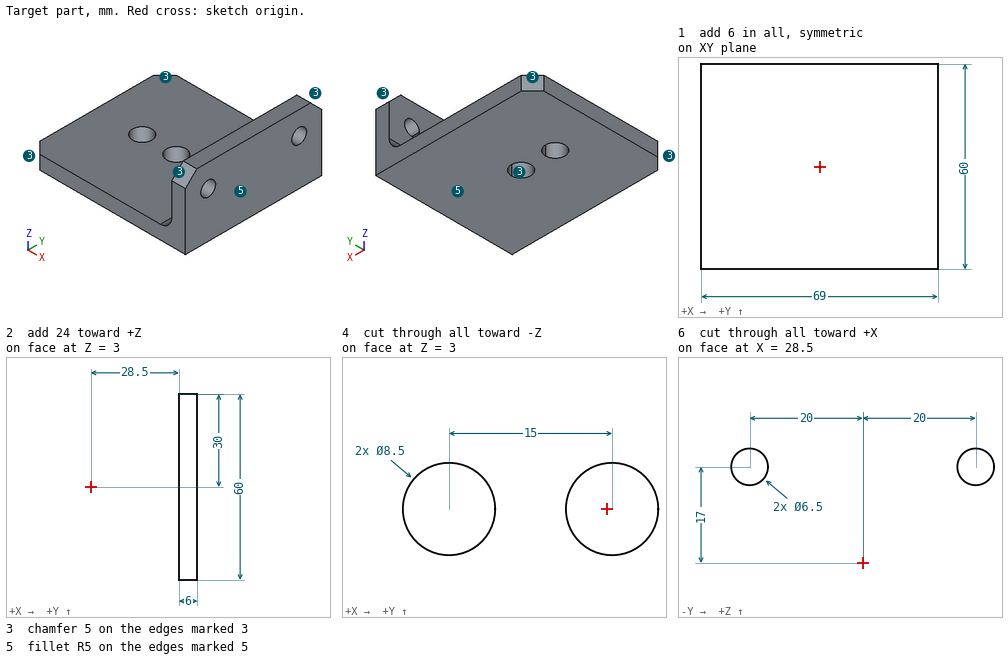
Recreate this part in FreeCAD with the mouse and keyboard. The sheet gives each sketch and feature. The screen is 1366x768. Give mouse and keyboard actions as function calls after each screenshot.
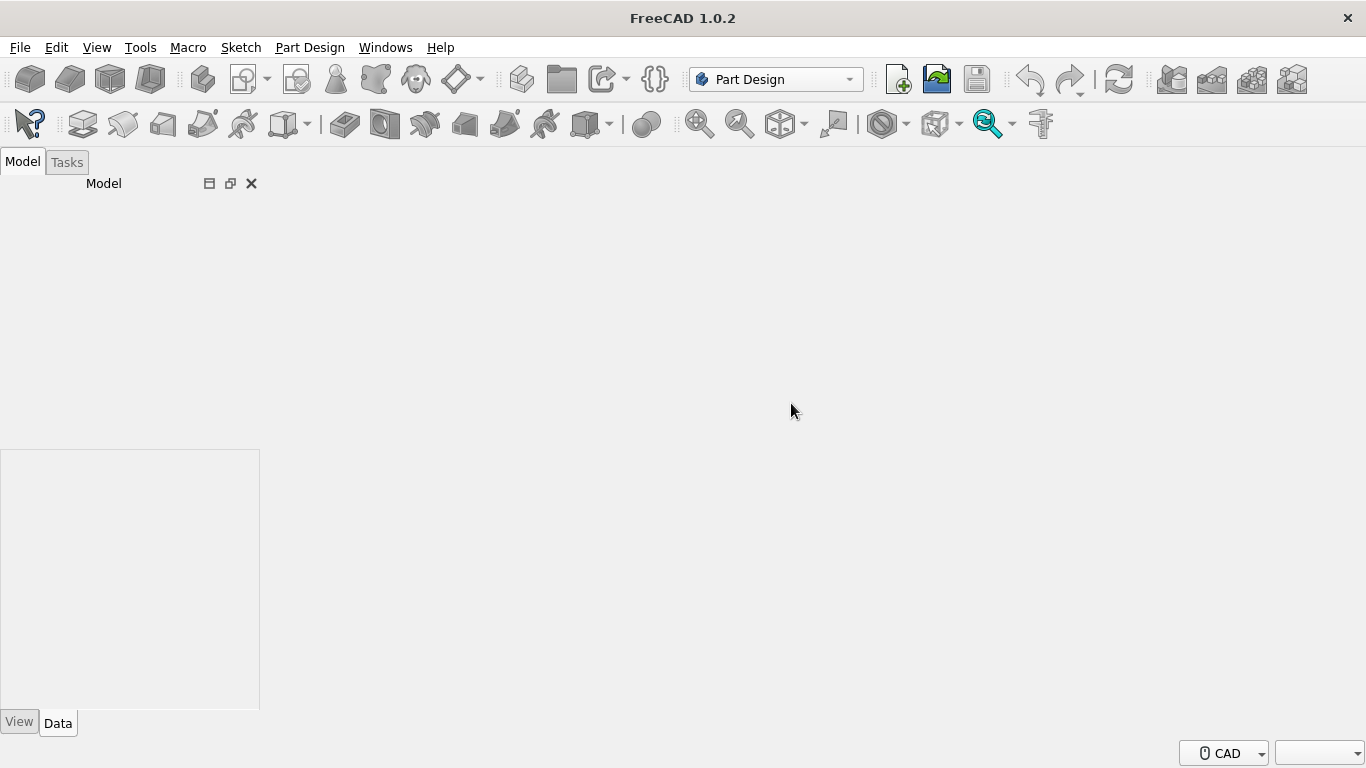
key(ctrl+n)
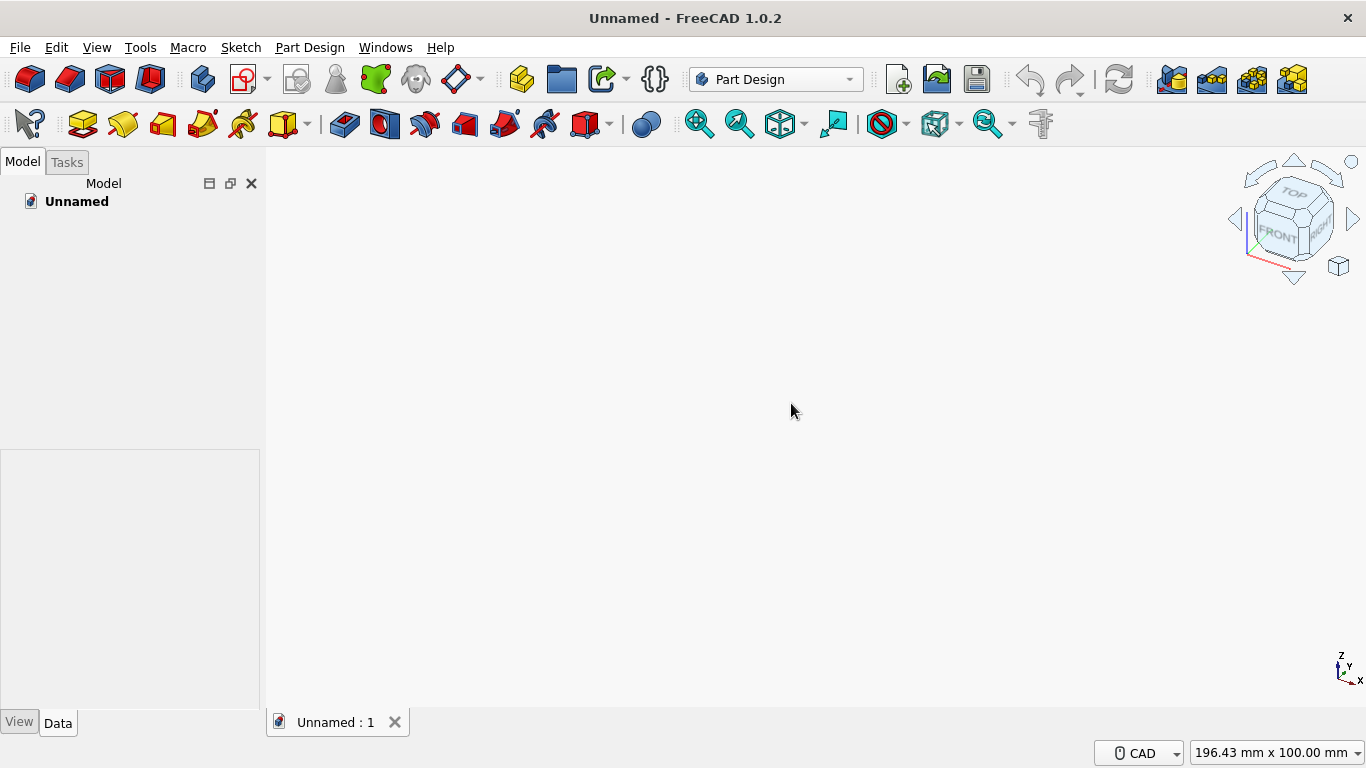
click(244, 80)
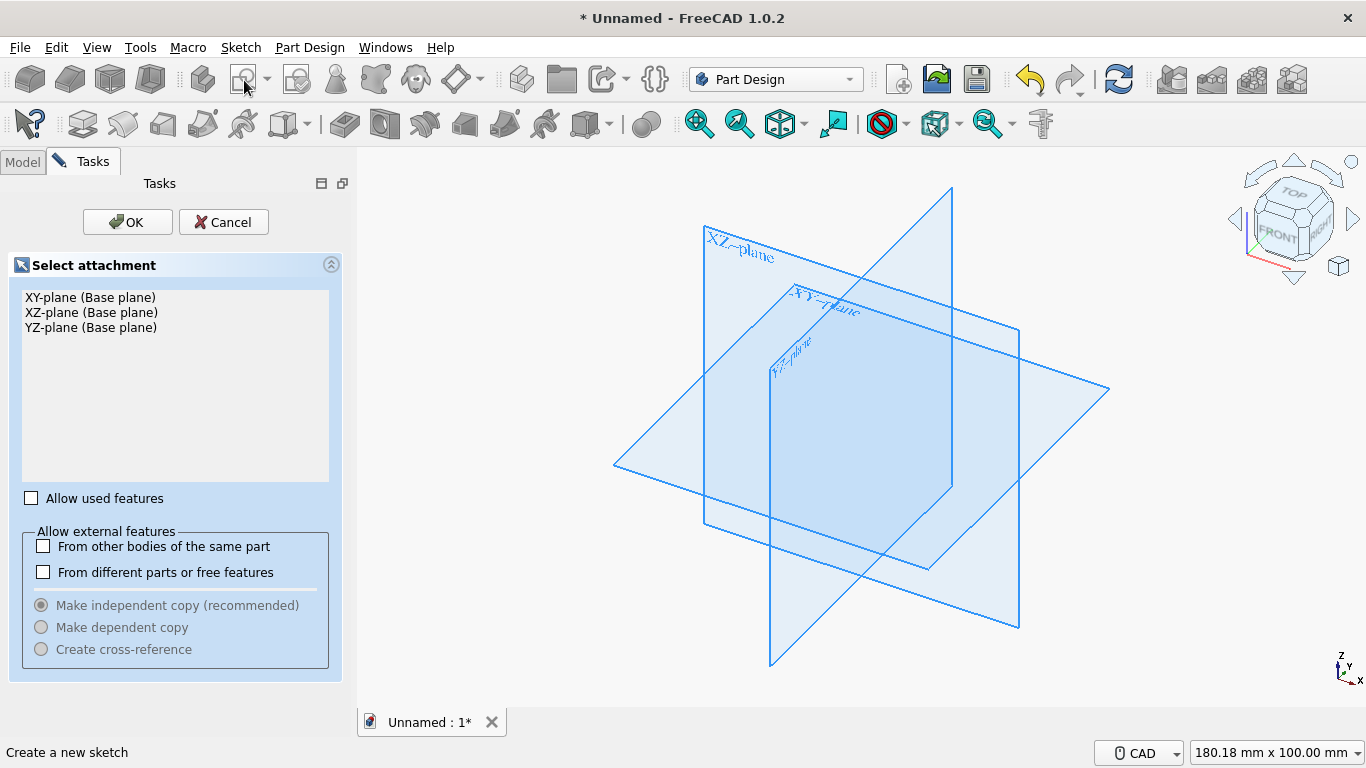
click(82, 298)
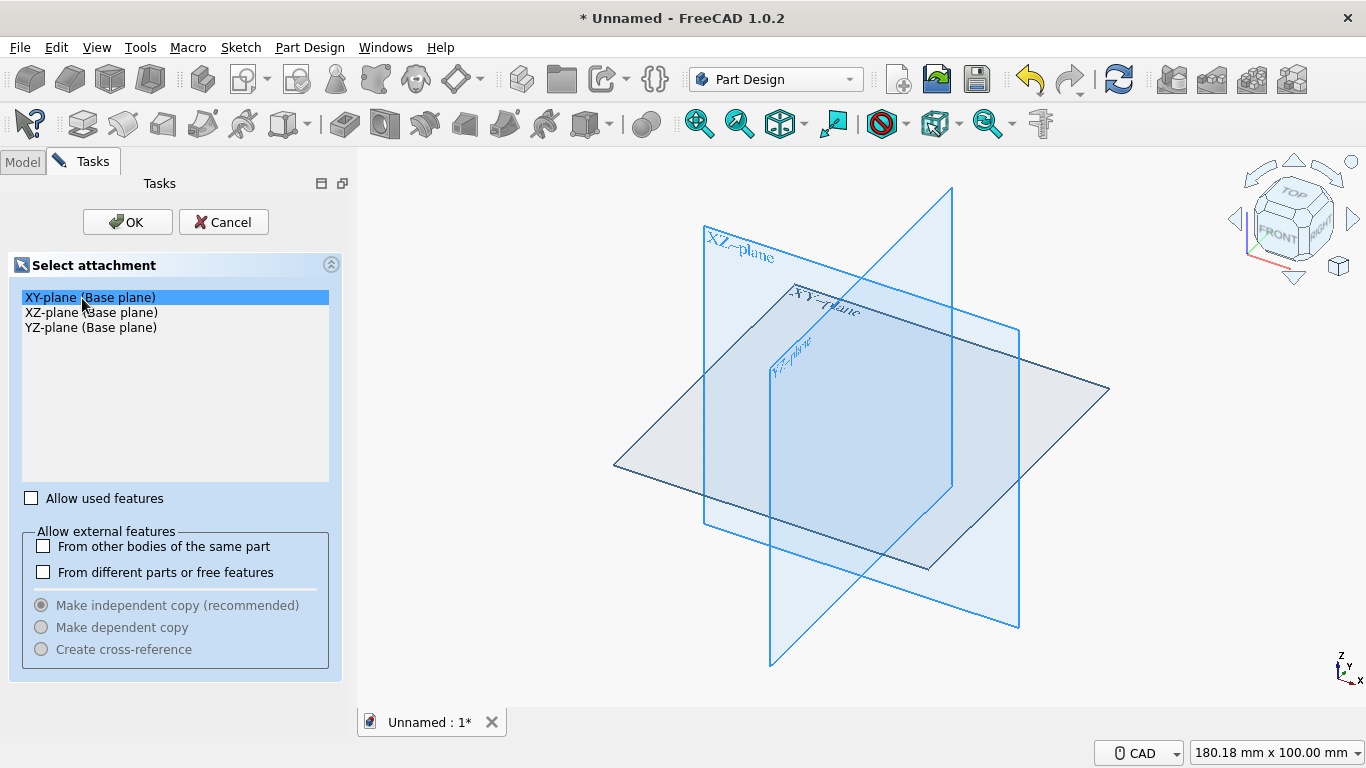
click(128, 222)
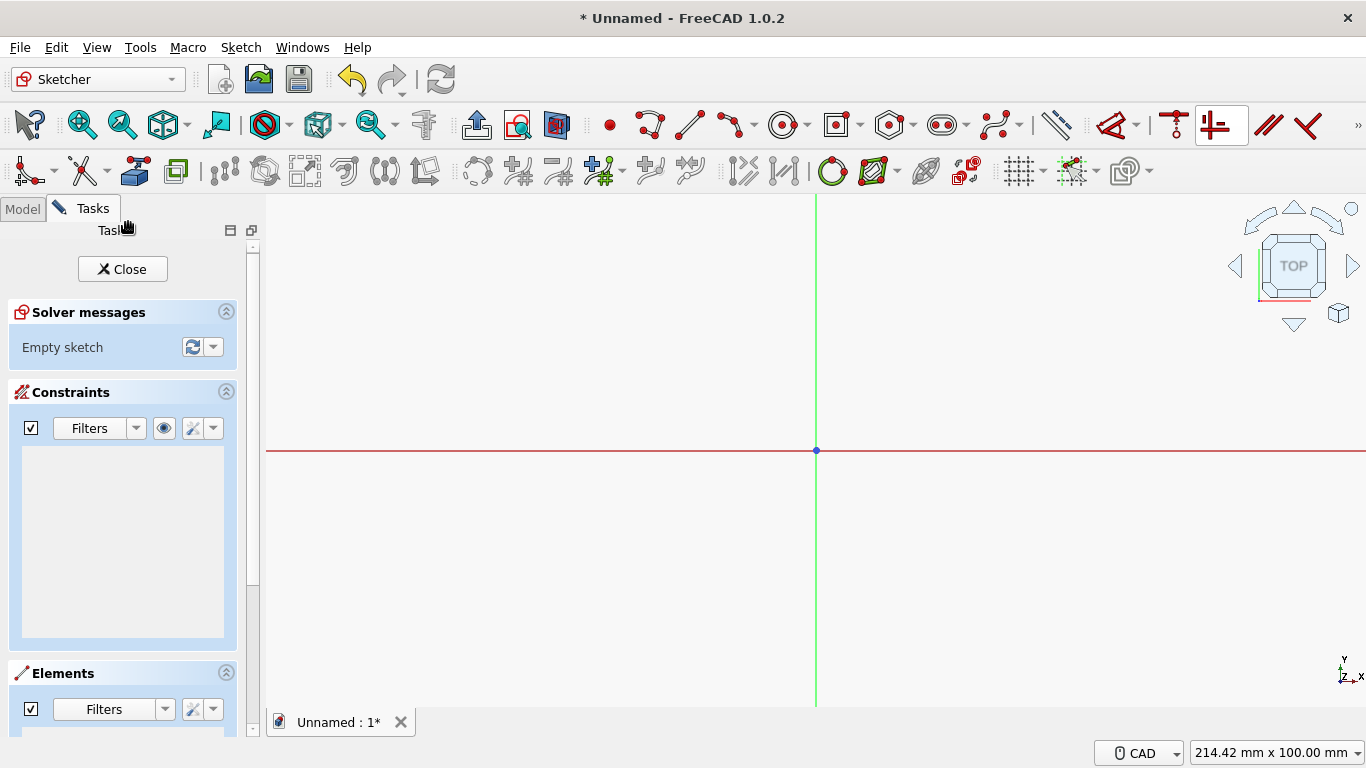
click(836, 126)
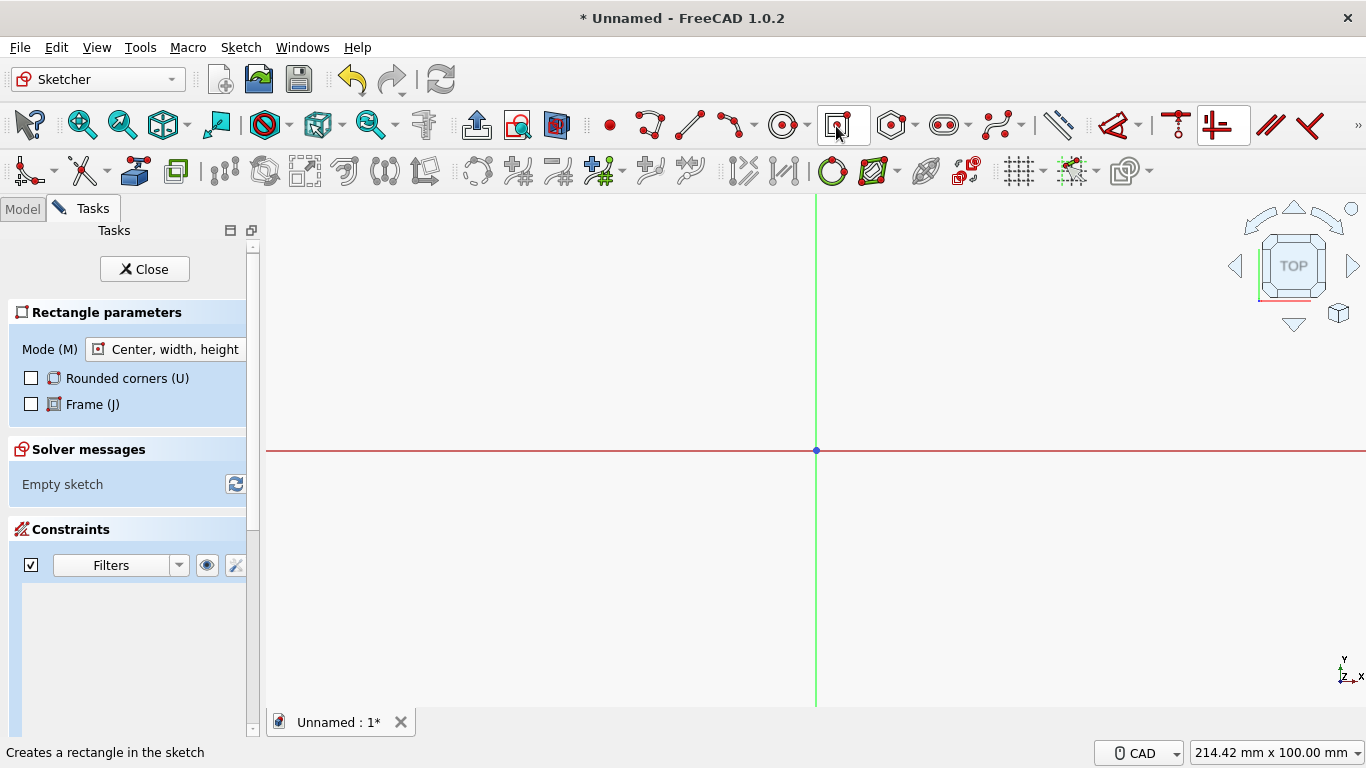
click(816, 450)
move(993, 297)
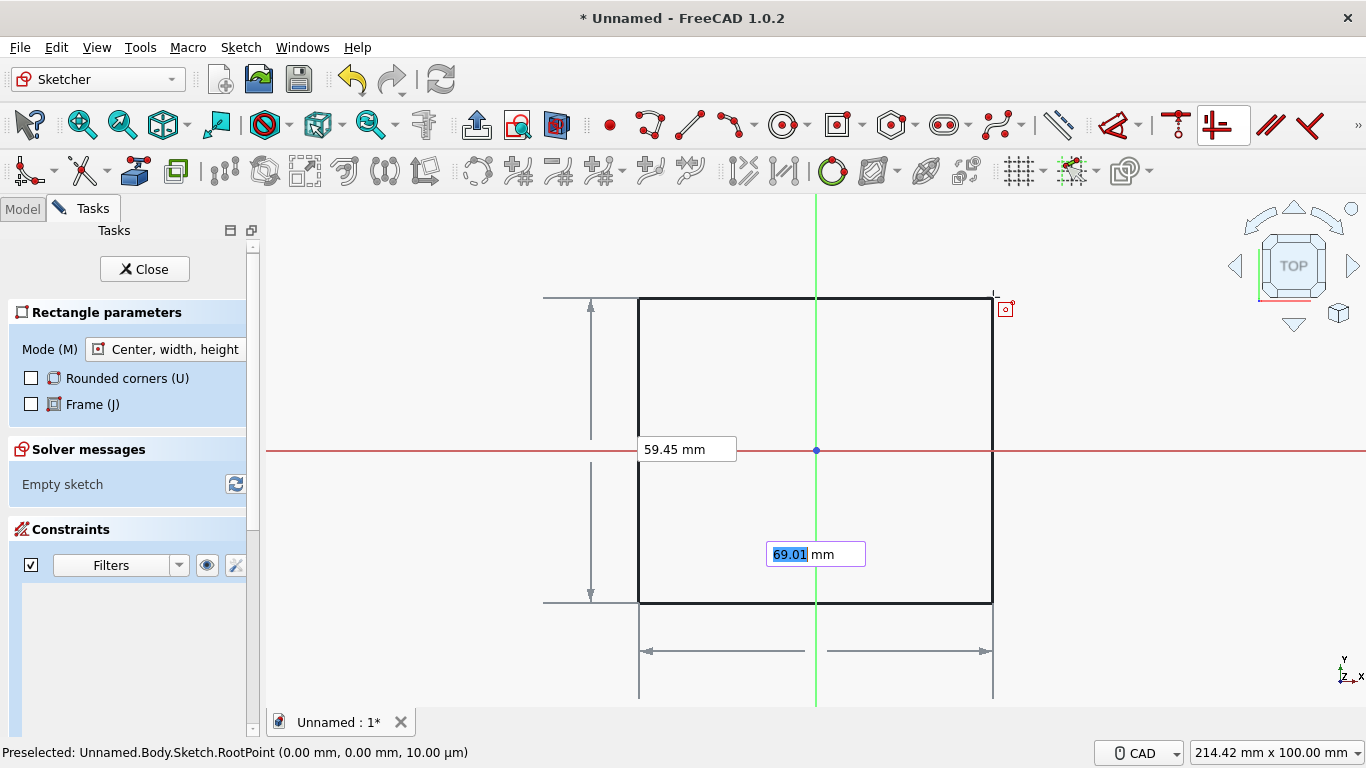
text(69)
key(Tab)
text(60)
key(Return)
key(Escape)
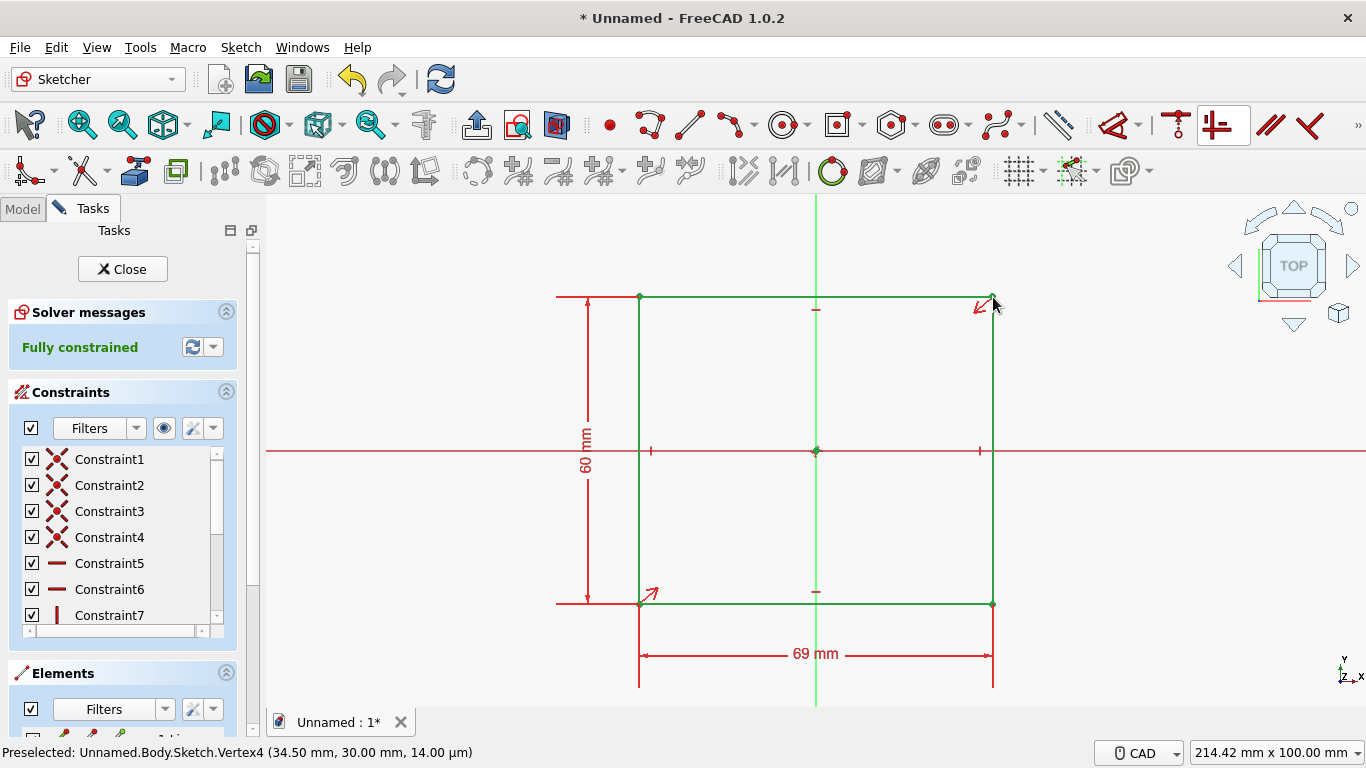
click(123, 269)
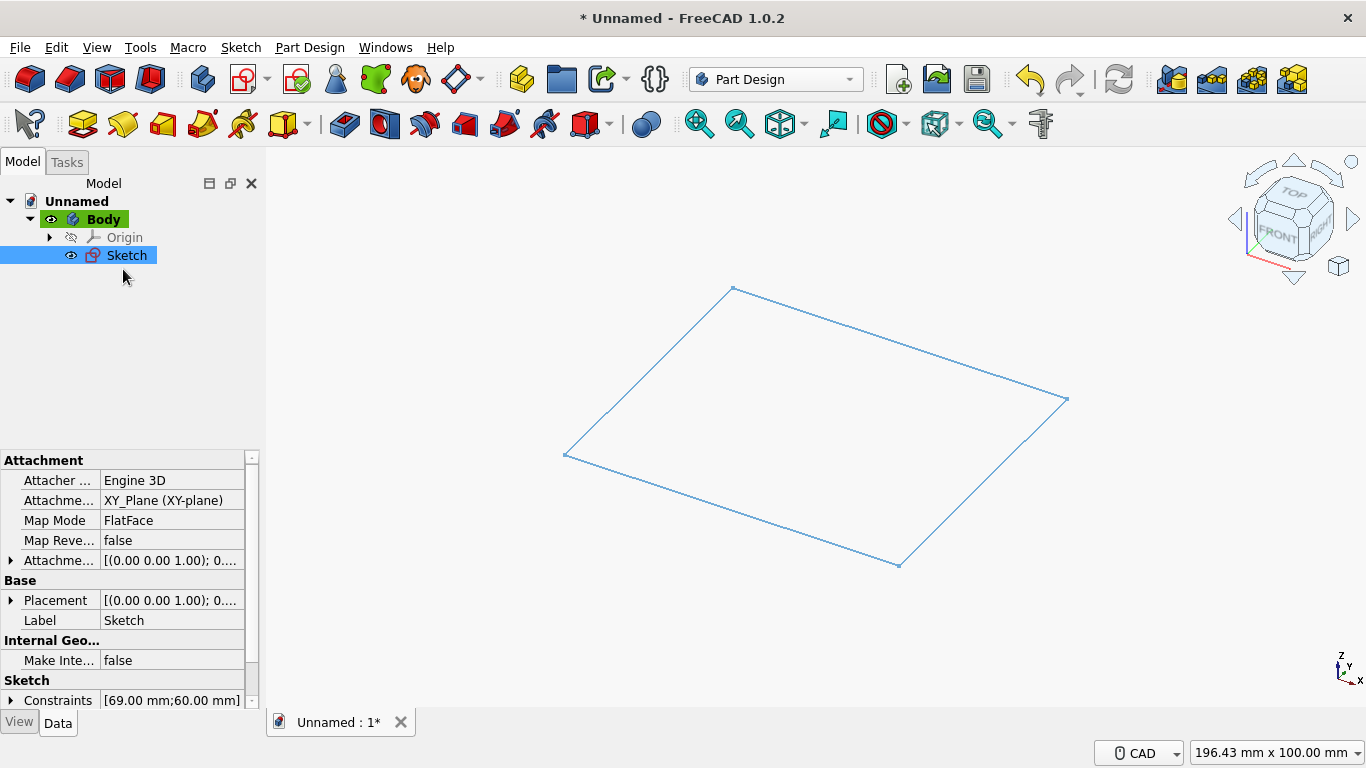
click(84, 124)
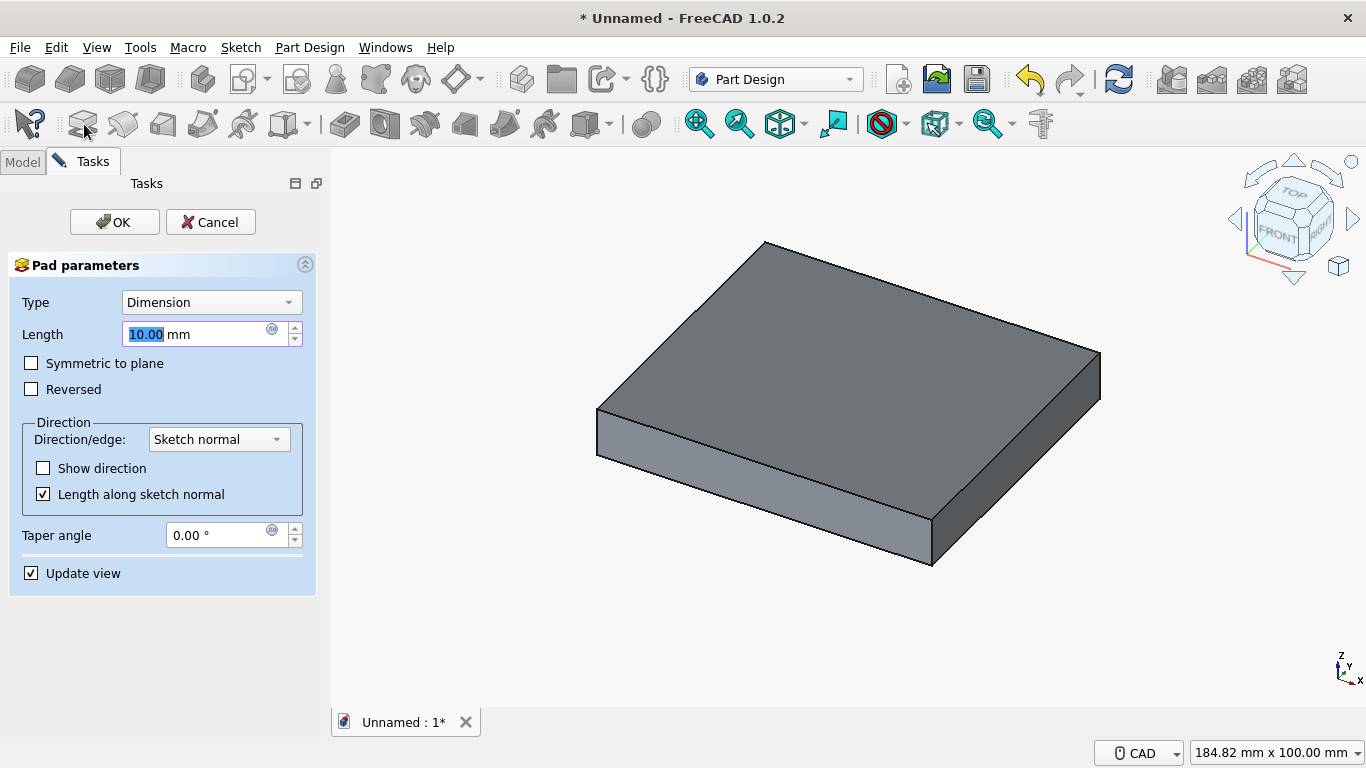
text(6)
key(Tab)